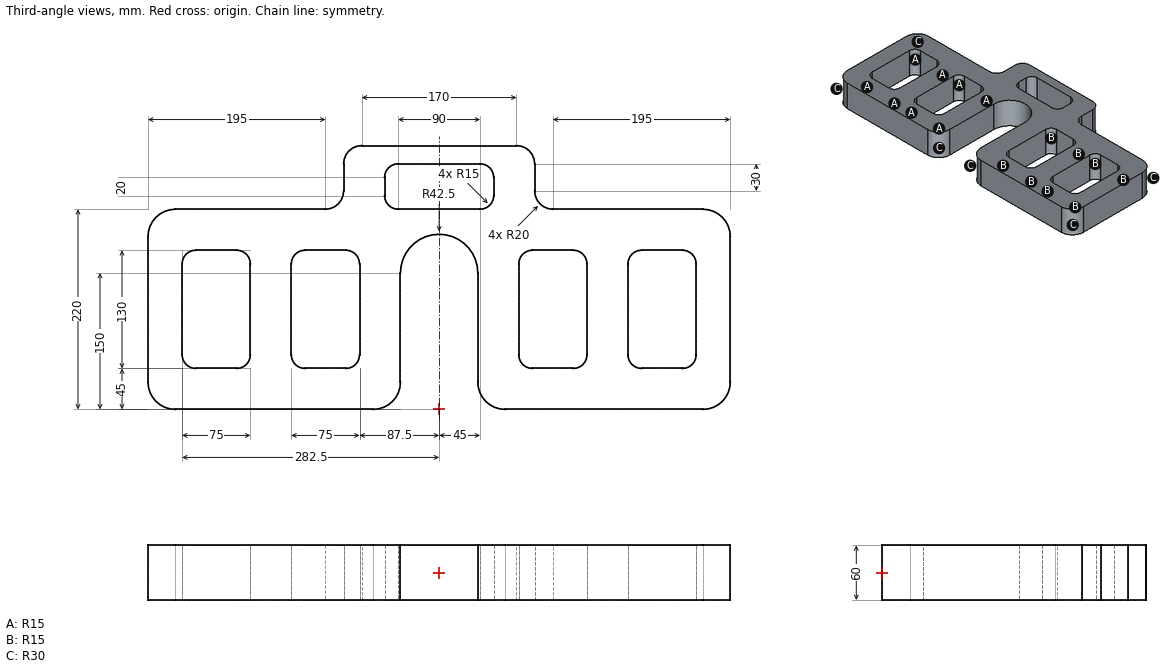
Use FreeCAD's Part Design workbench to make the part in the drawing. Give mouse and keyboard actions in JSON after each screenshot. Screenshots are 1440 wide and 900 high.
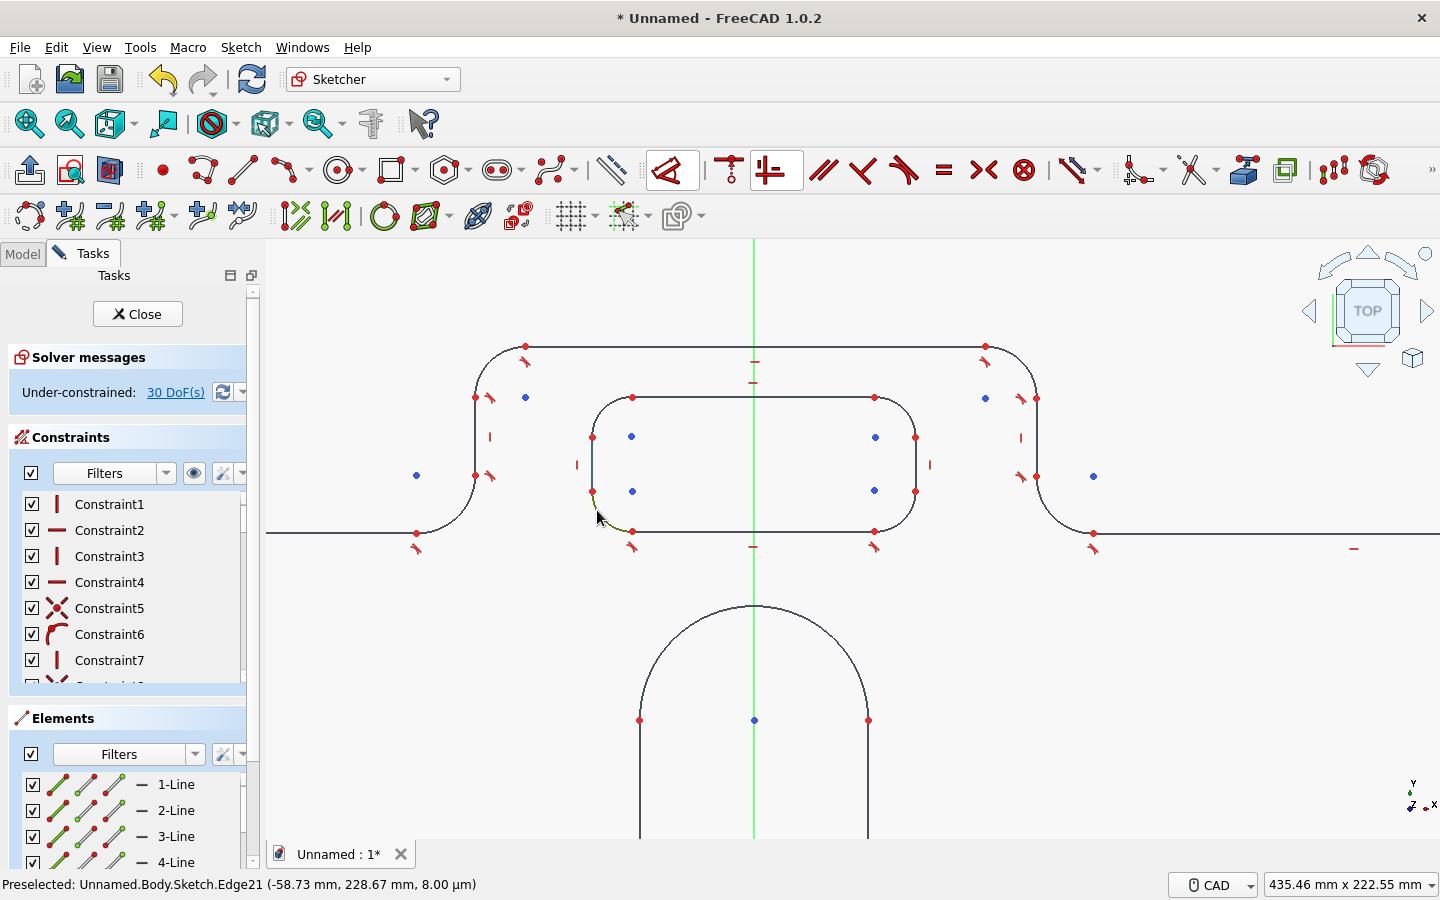
{"action": "key", "text": "t"}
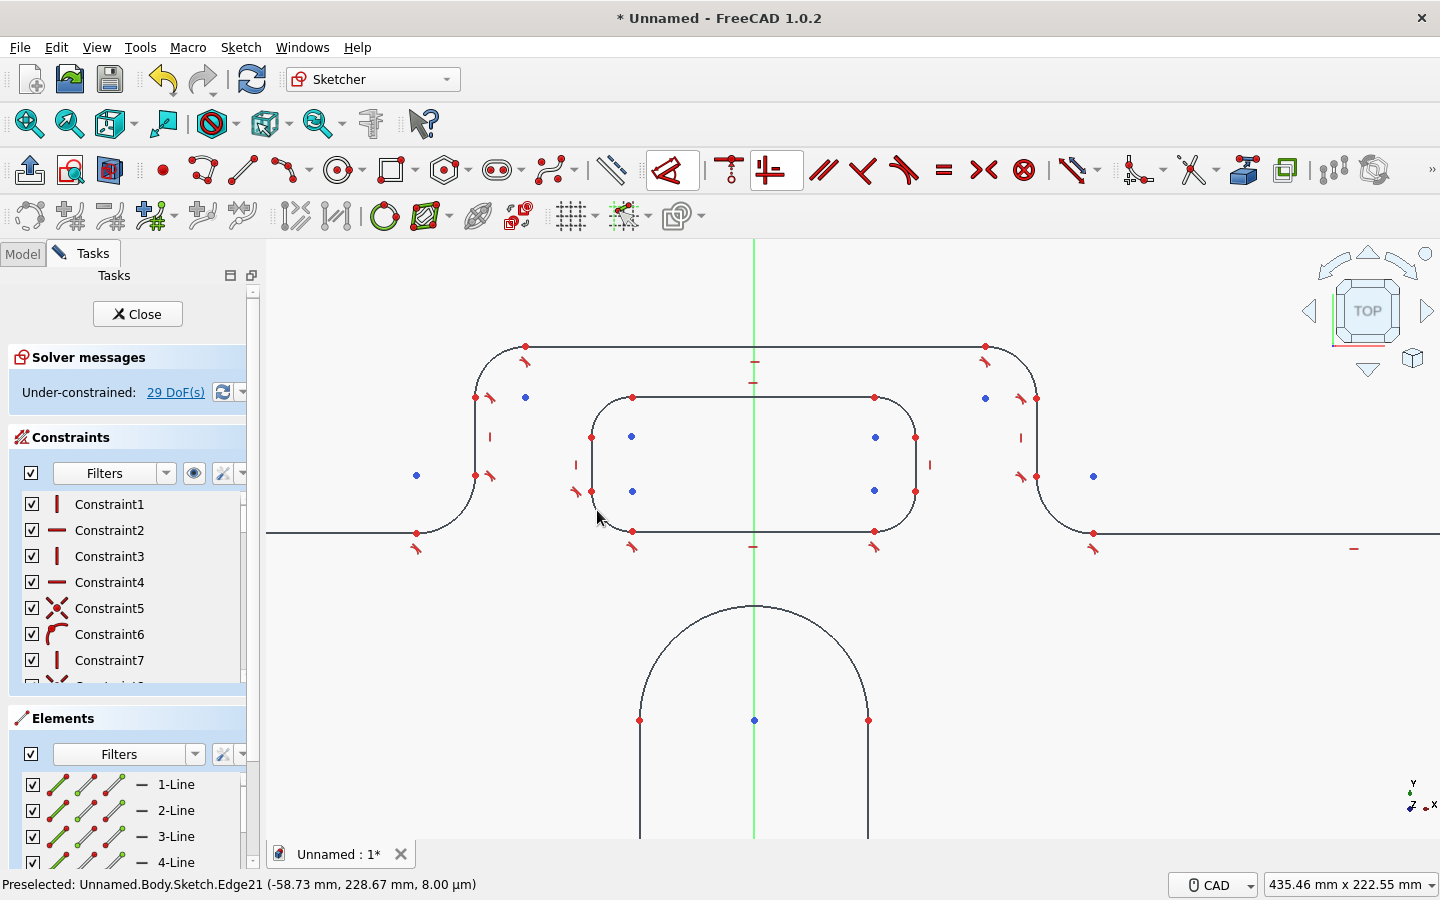
{"action": "left_click", "coordinate": [592, 475]}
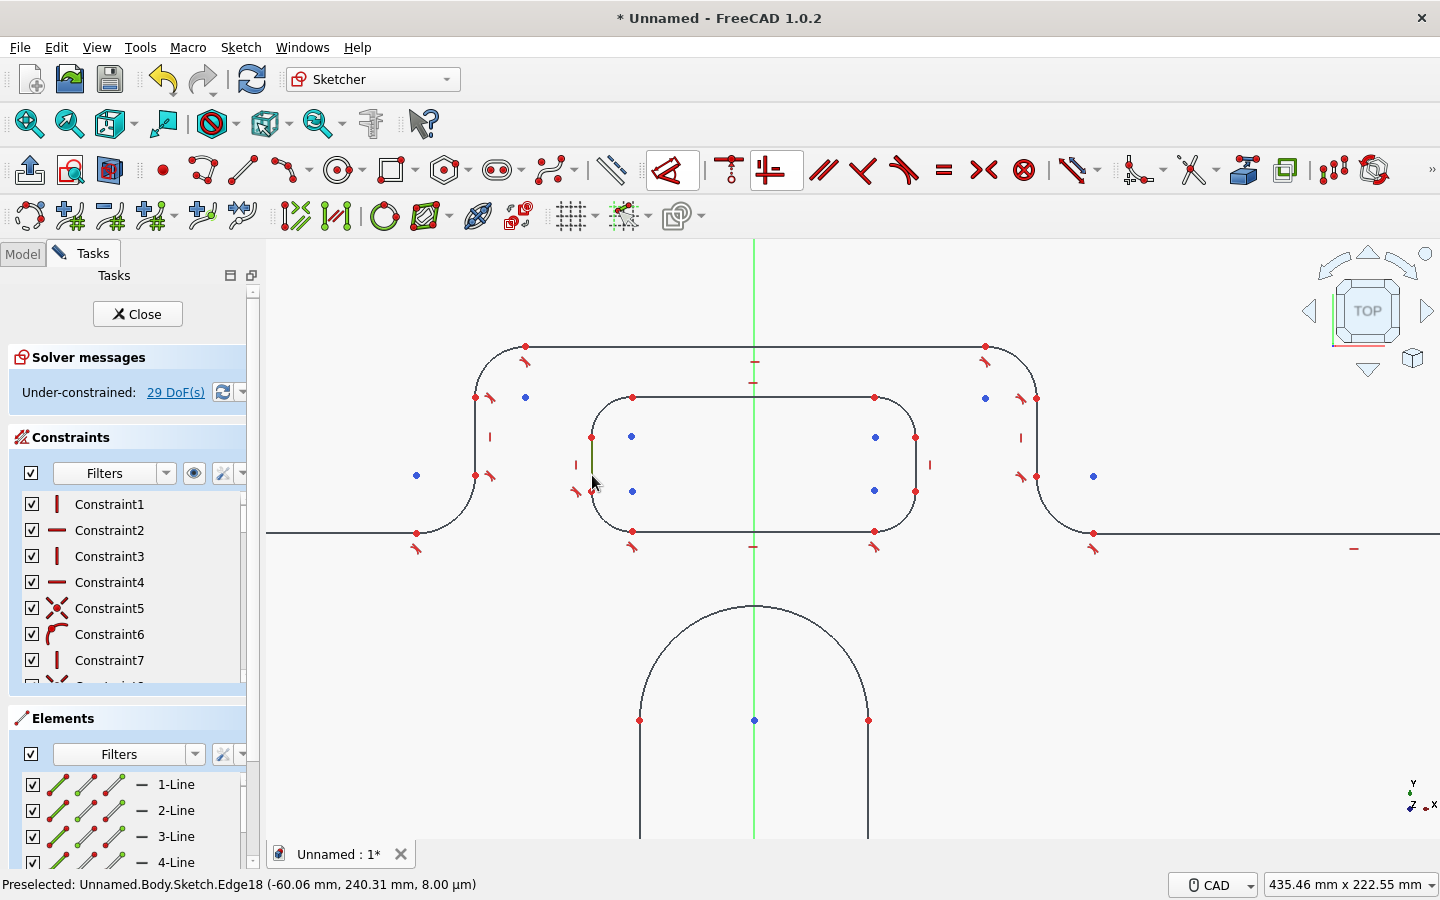
{"action": "left_click", "coordinate": [614, 401]}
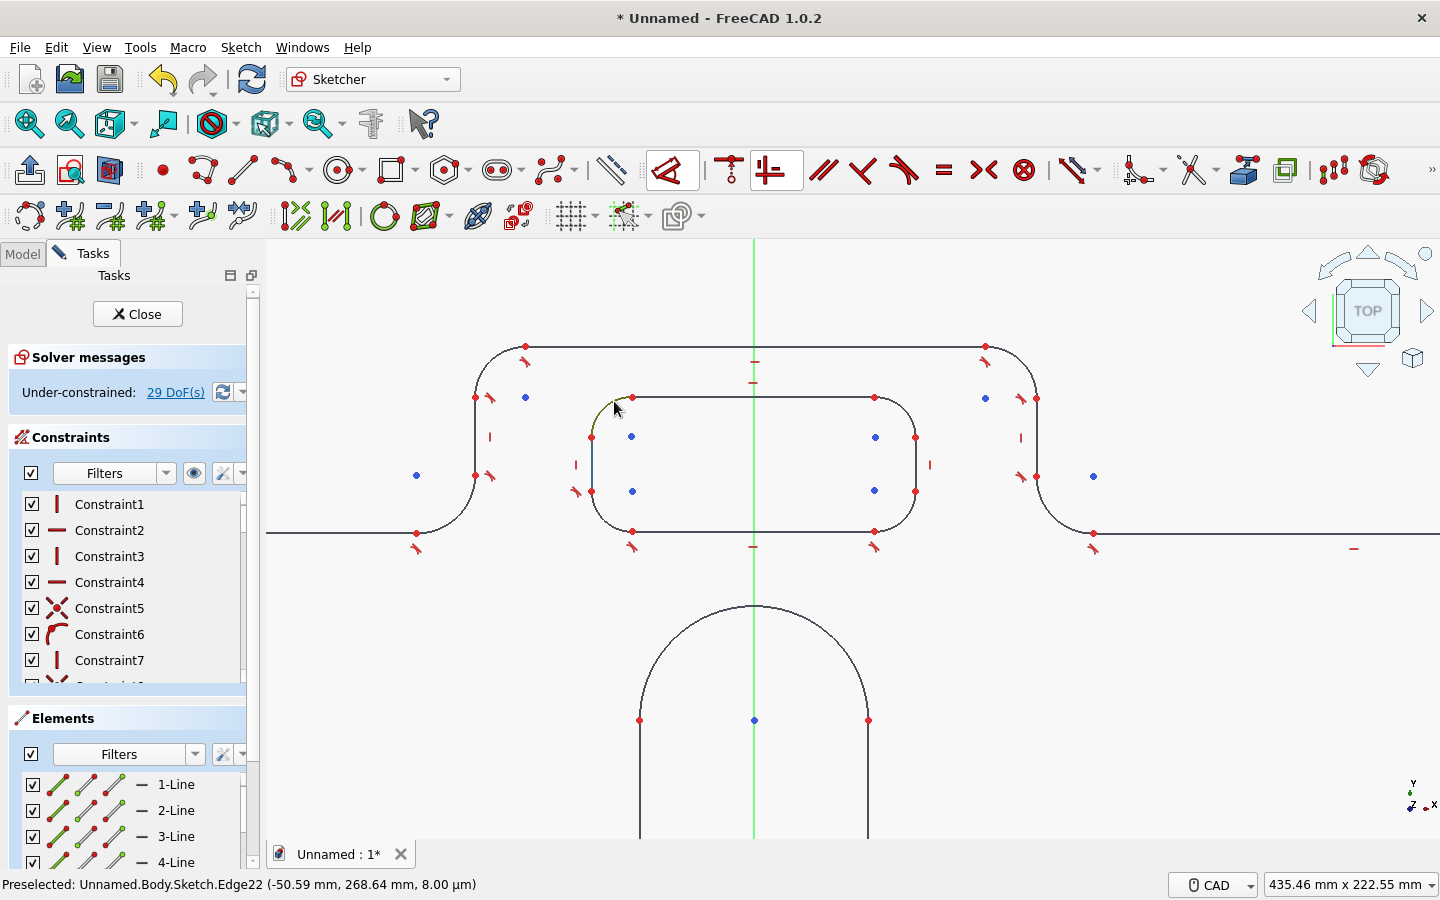
{"action": "key", "text": "t"}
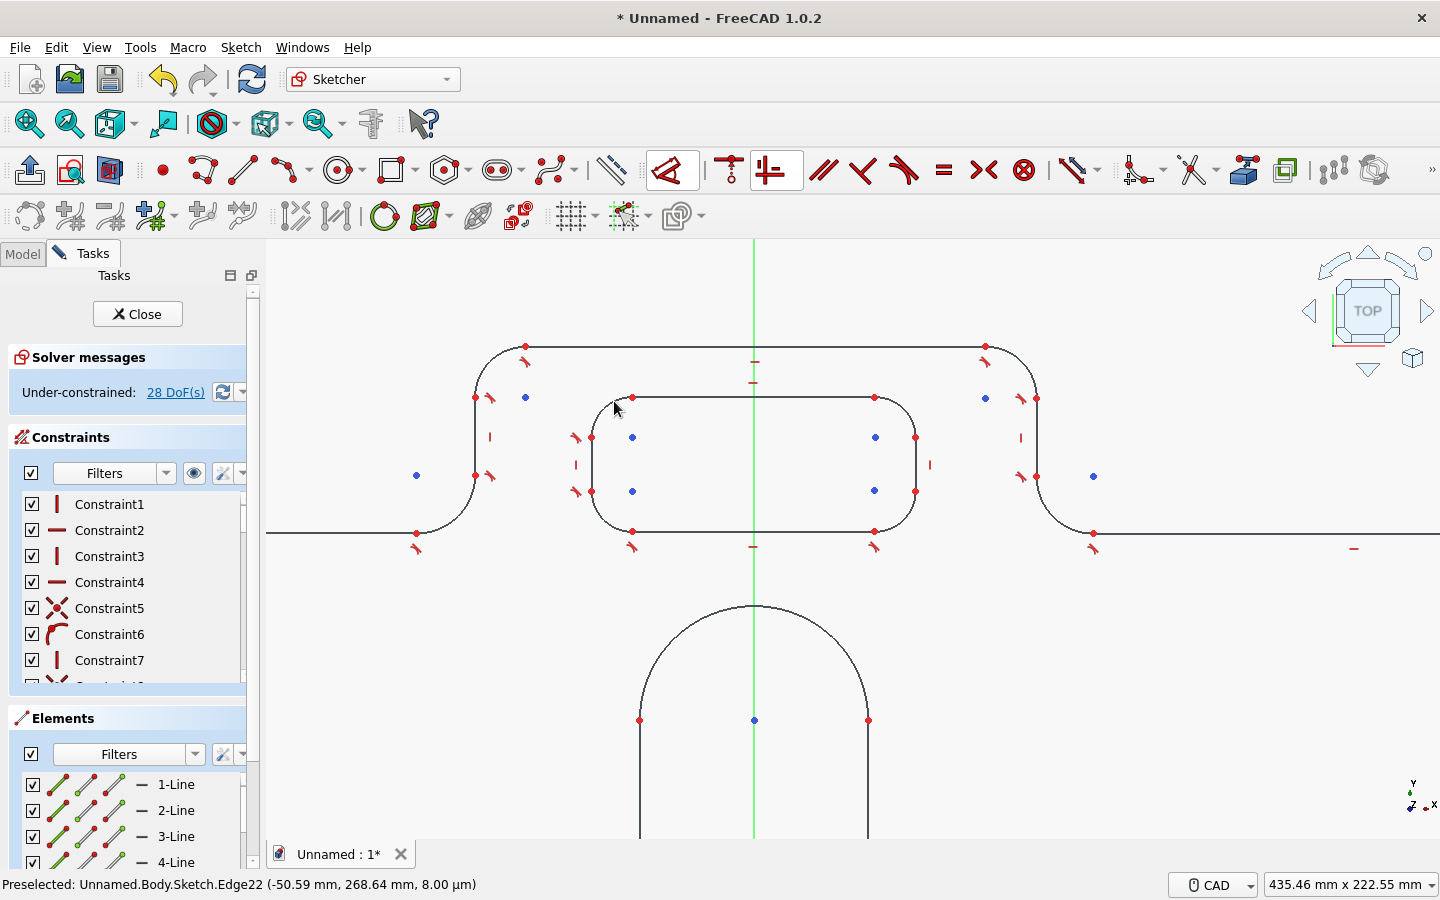
{"action": "left_click", "coordinate": [705, 397]}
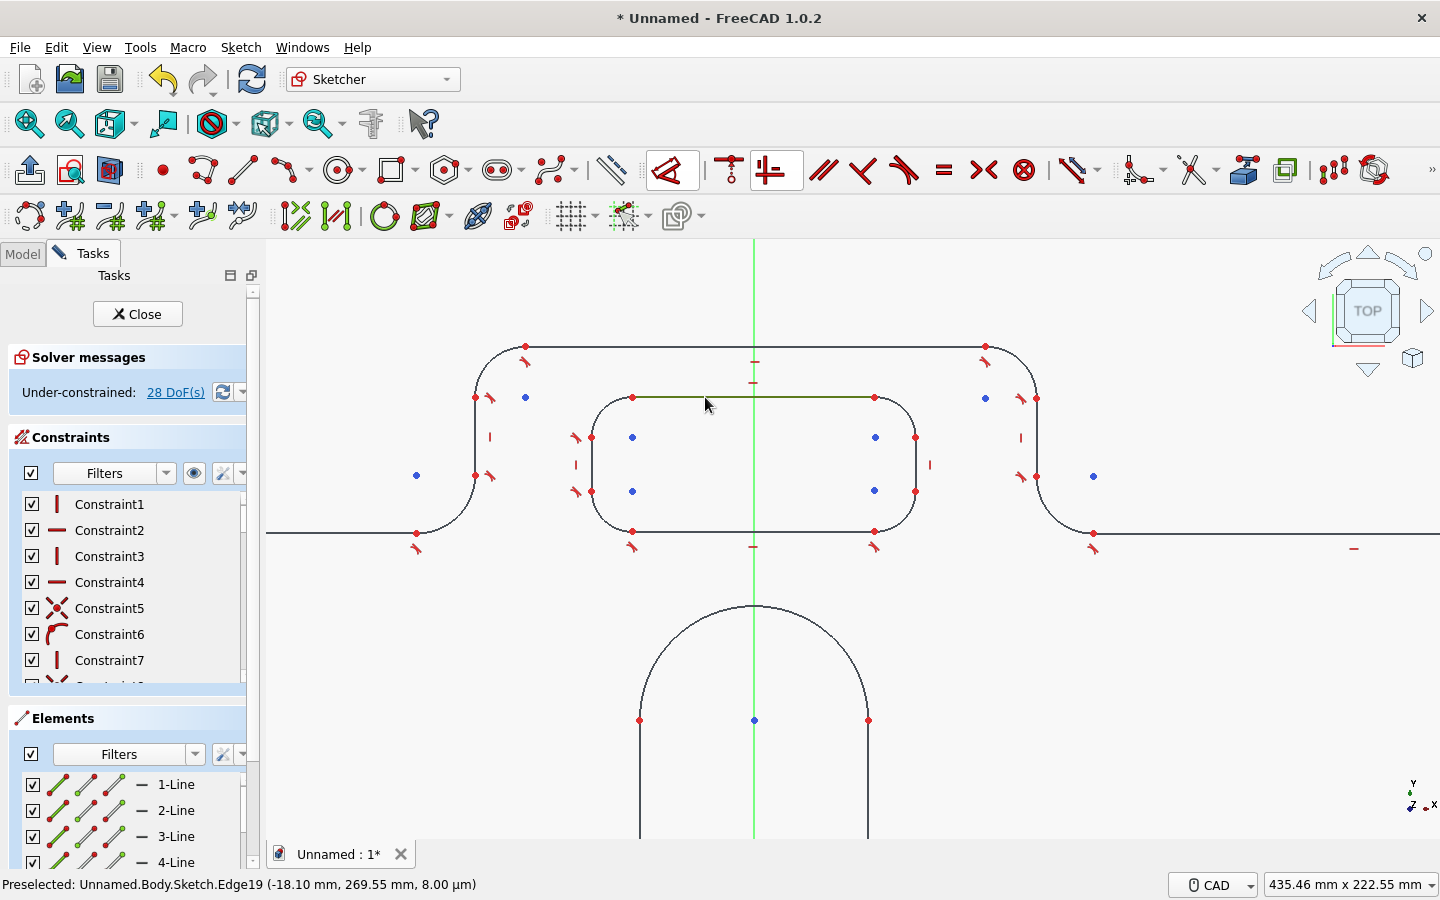
{"action": "left_click", "coordinate": [614, 401]}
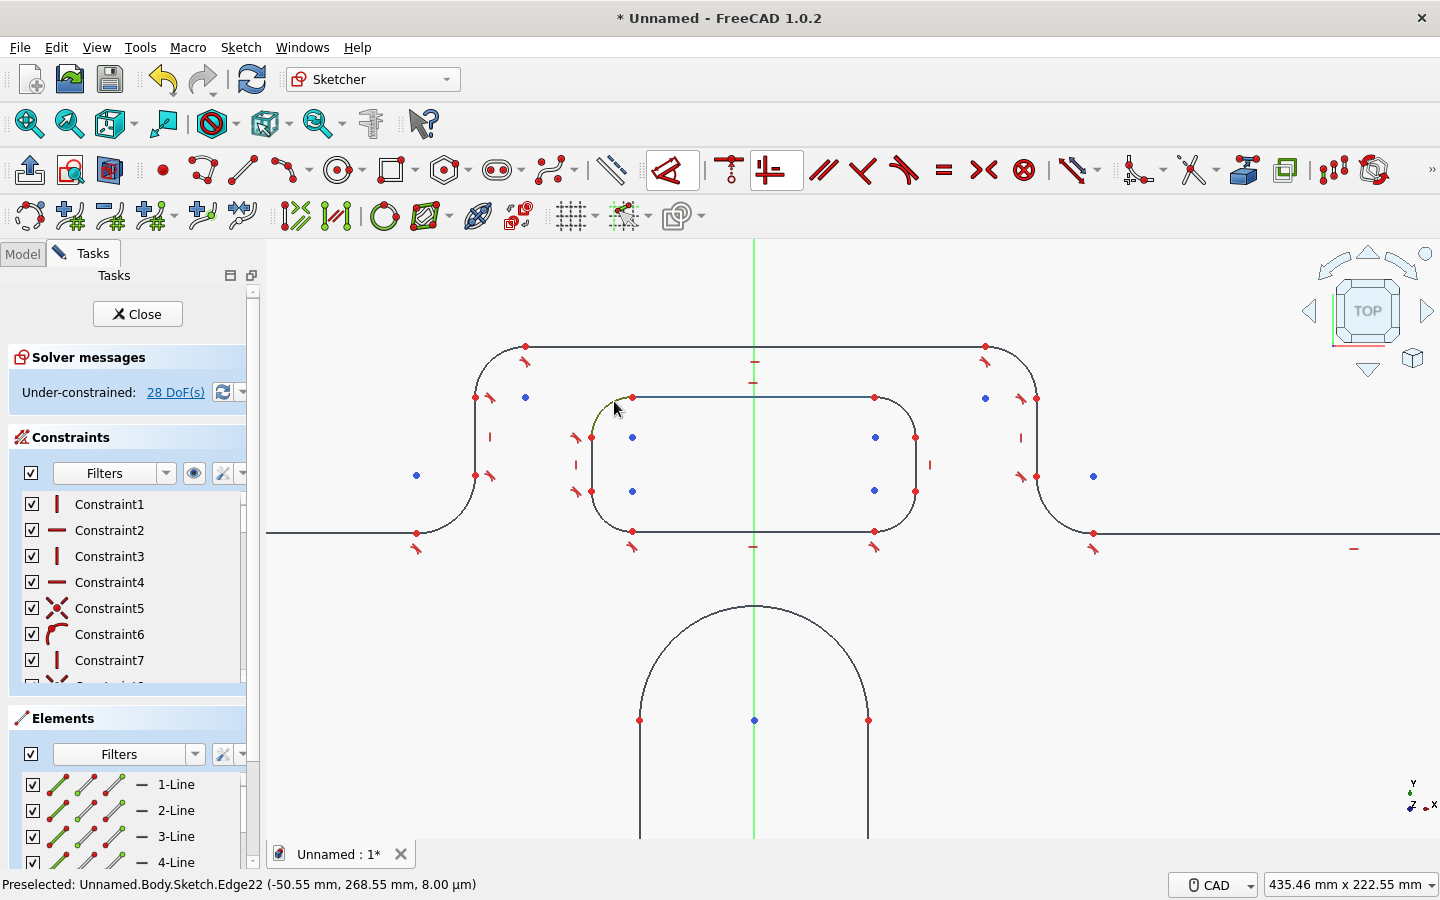
{"action": "left_click", "coordinate": [904, 170]}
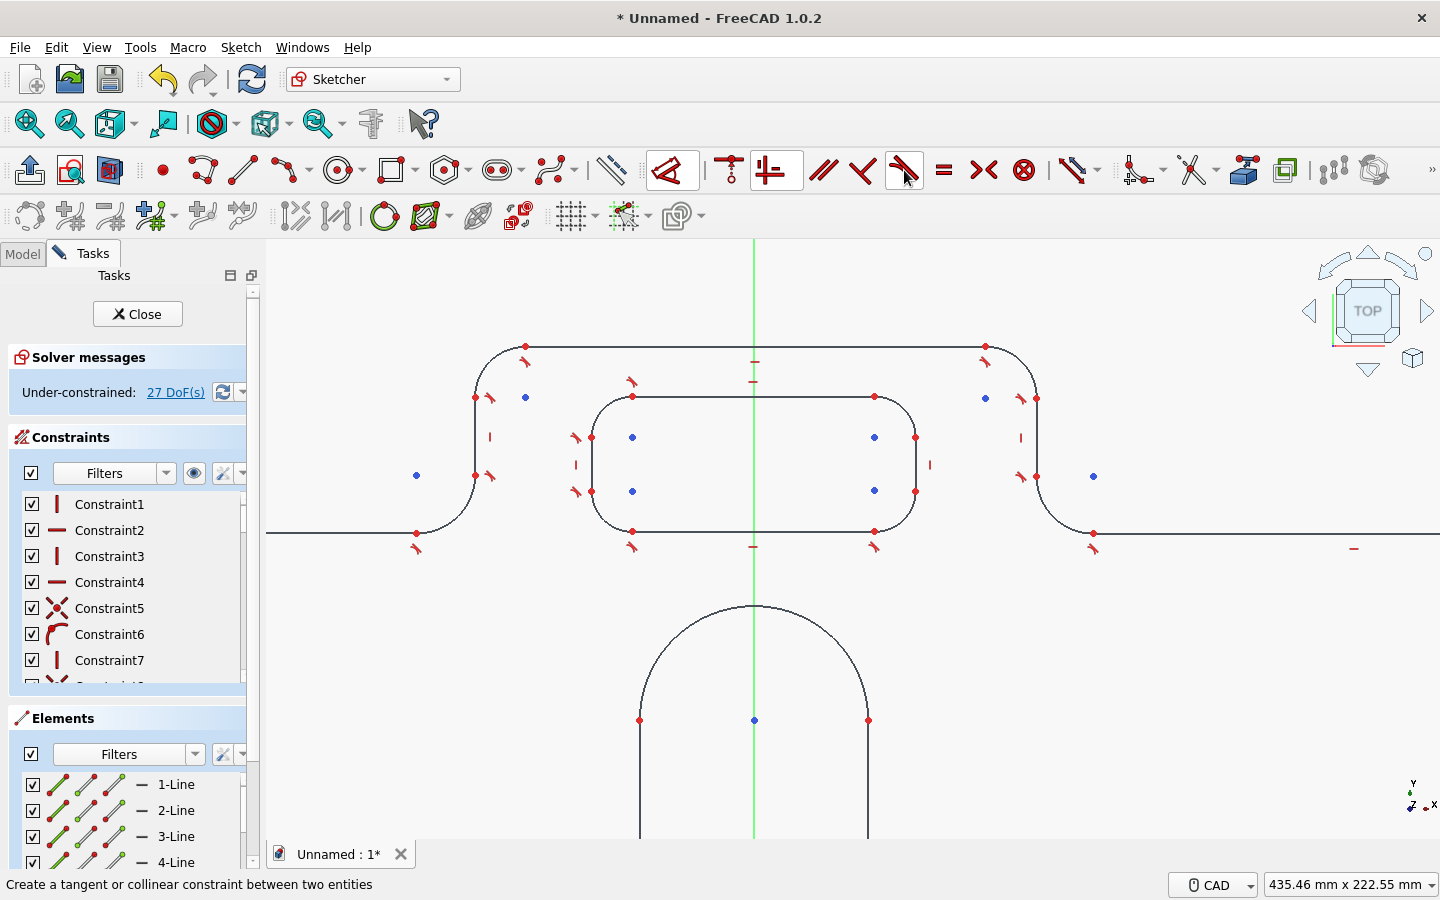
{"action": "left_click", "coordinate": [705, 397]}